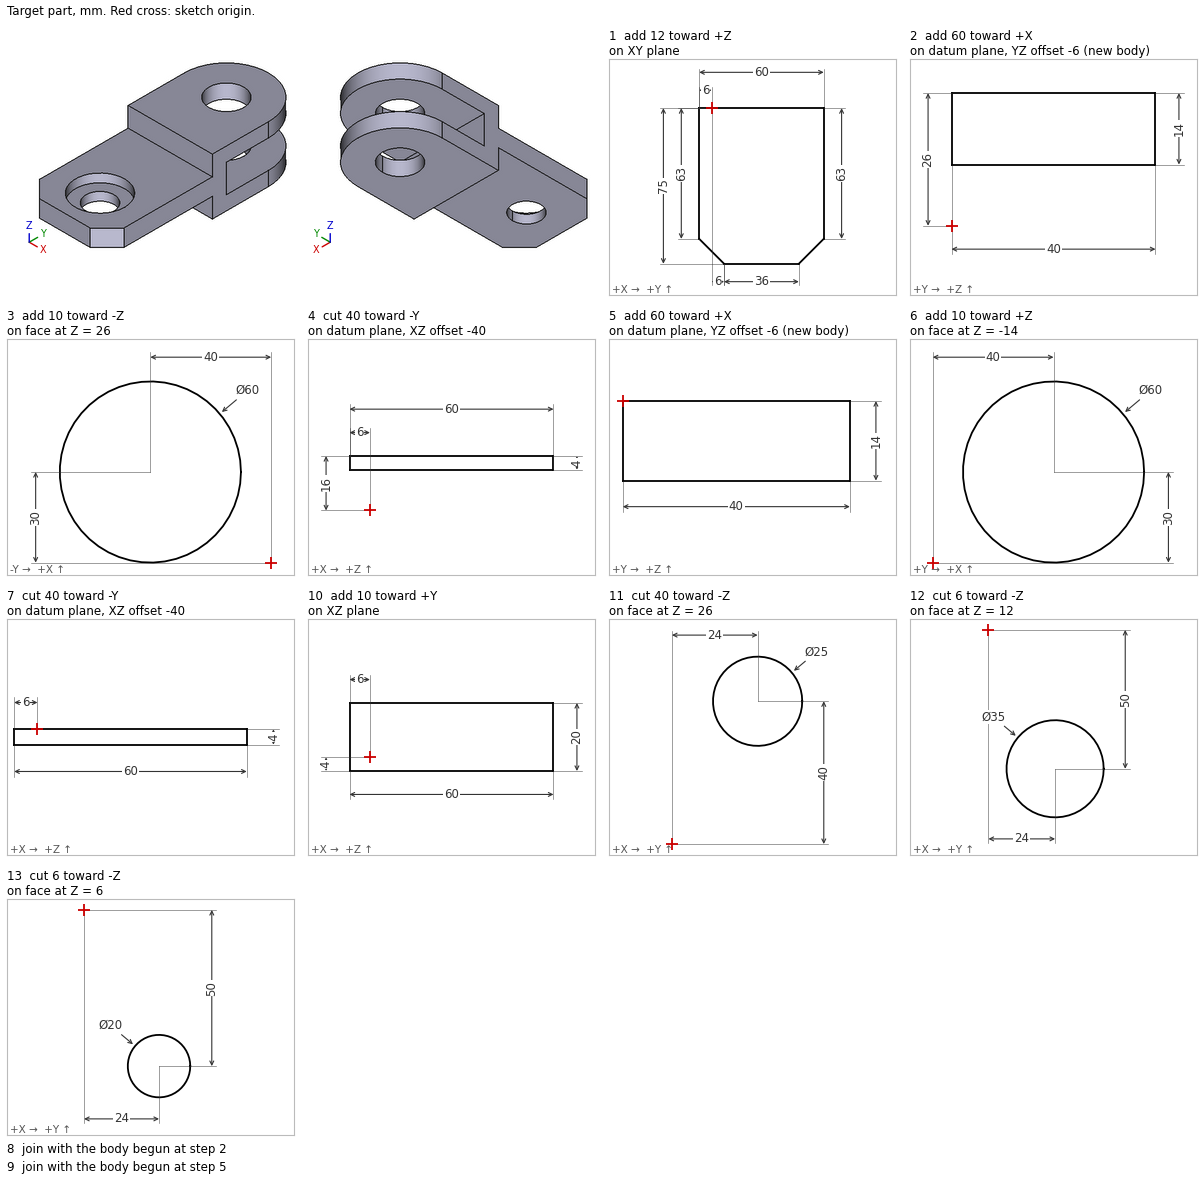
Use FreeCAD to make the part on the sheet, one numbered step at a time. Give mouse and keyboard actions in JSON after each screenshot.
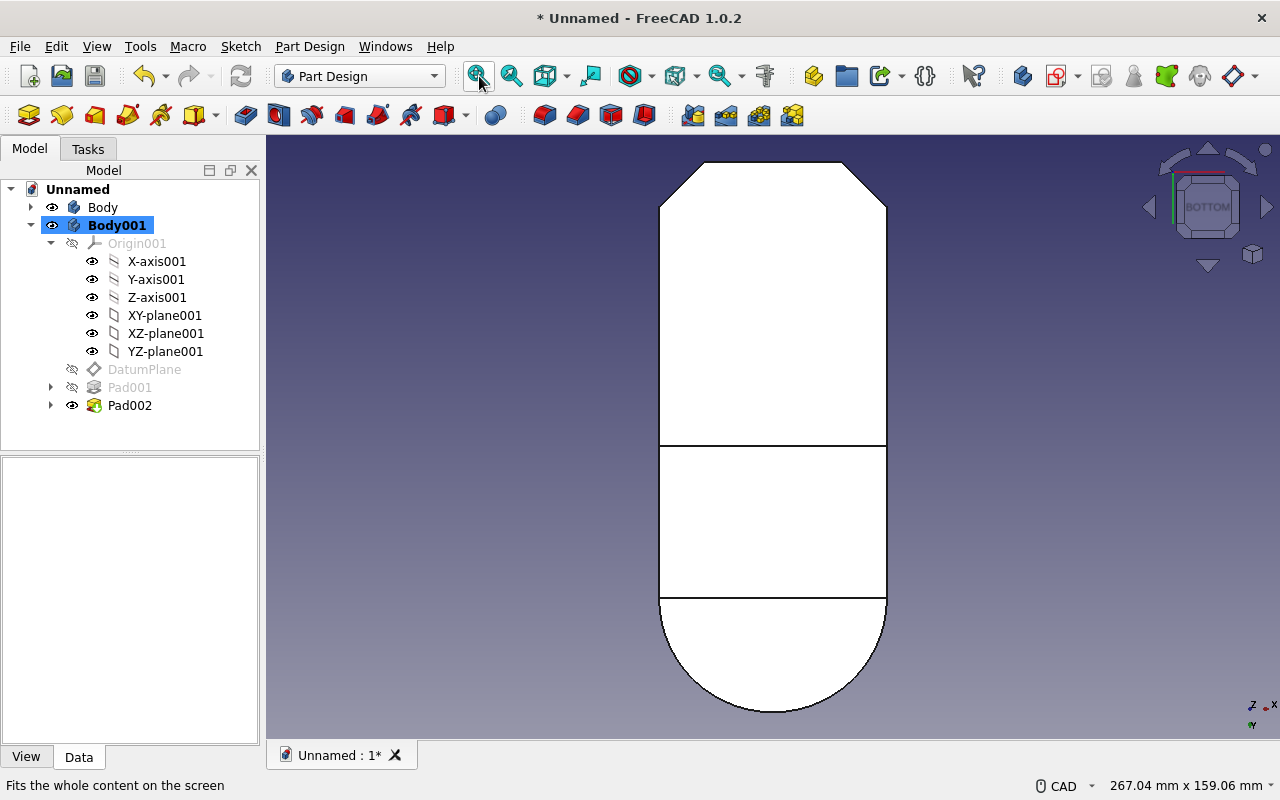
{"action": "key", "text": "3"}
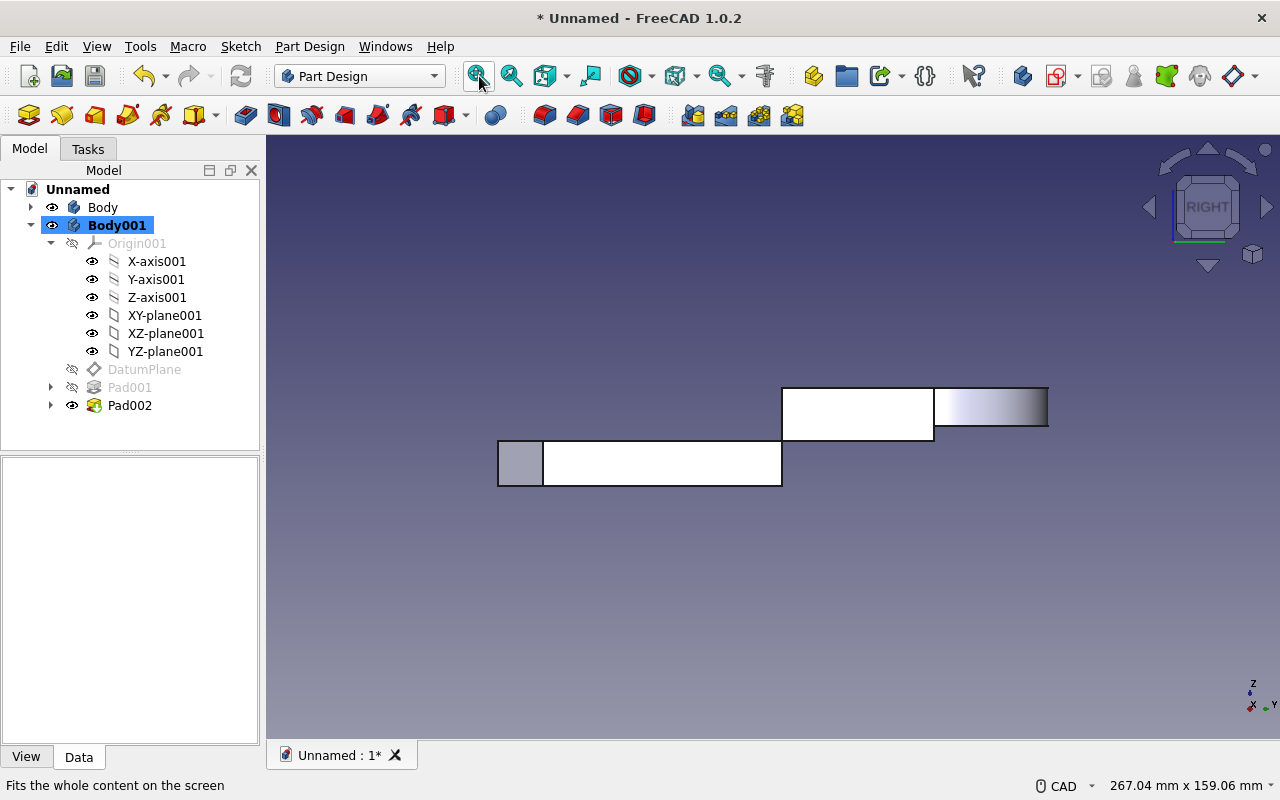
{"action": "left_click", "coordinate": [479, 76]}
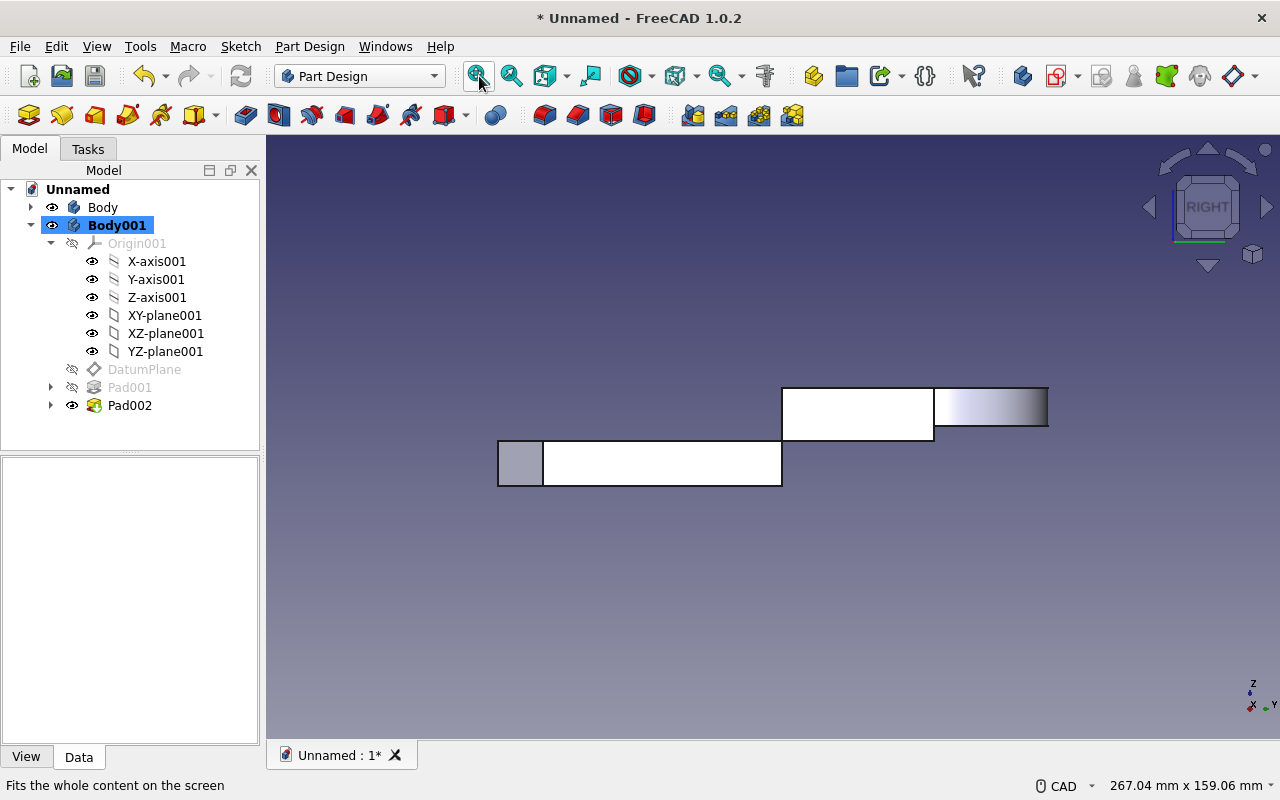
{"action": "left_click", "coordinate": [137, 333]}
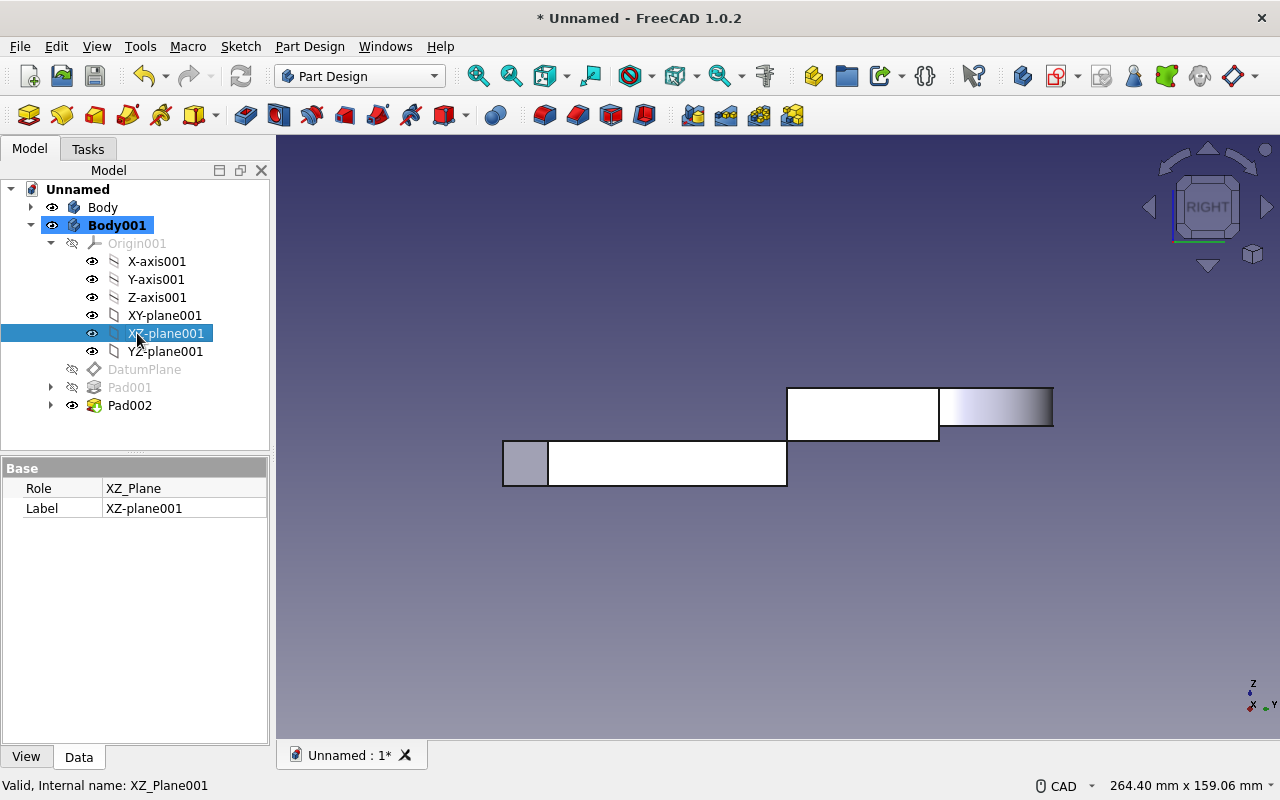
{"action": "left_click", "coordinate": [1232, 76]}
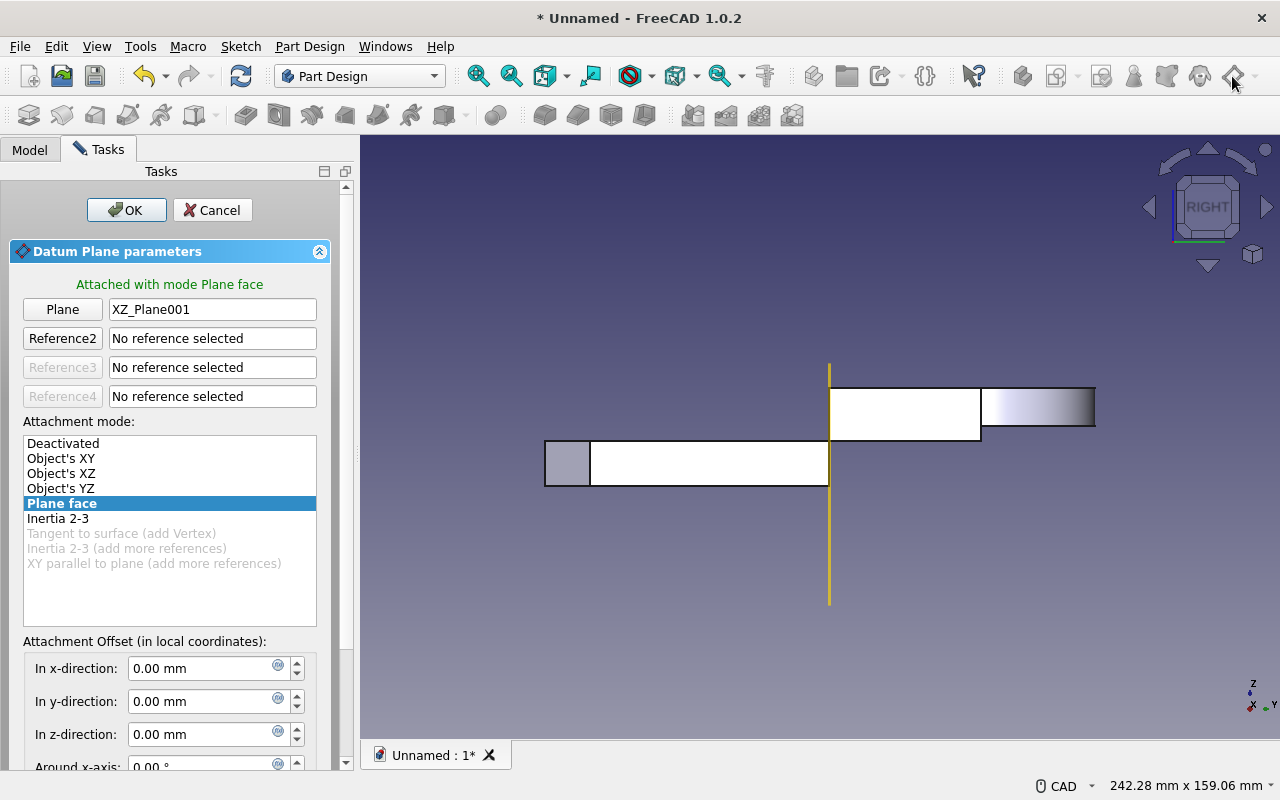
{"action": "triple_click", "coordinate": [210, 734]}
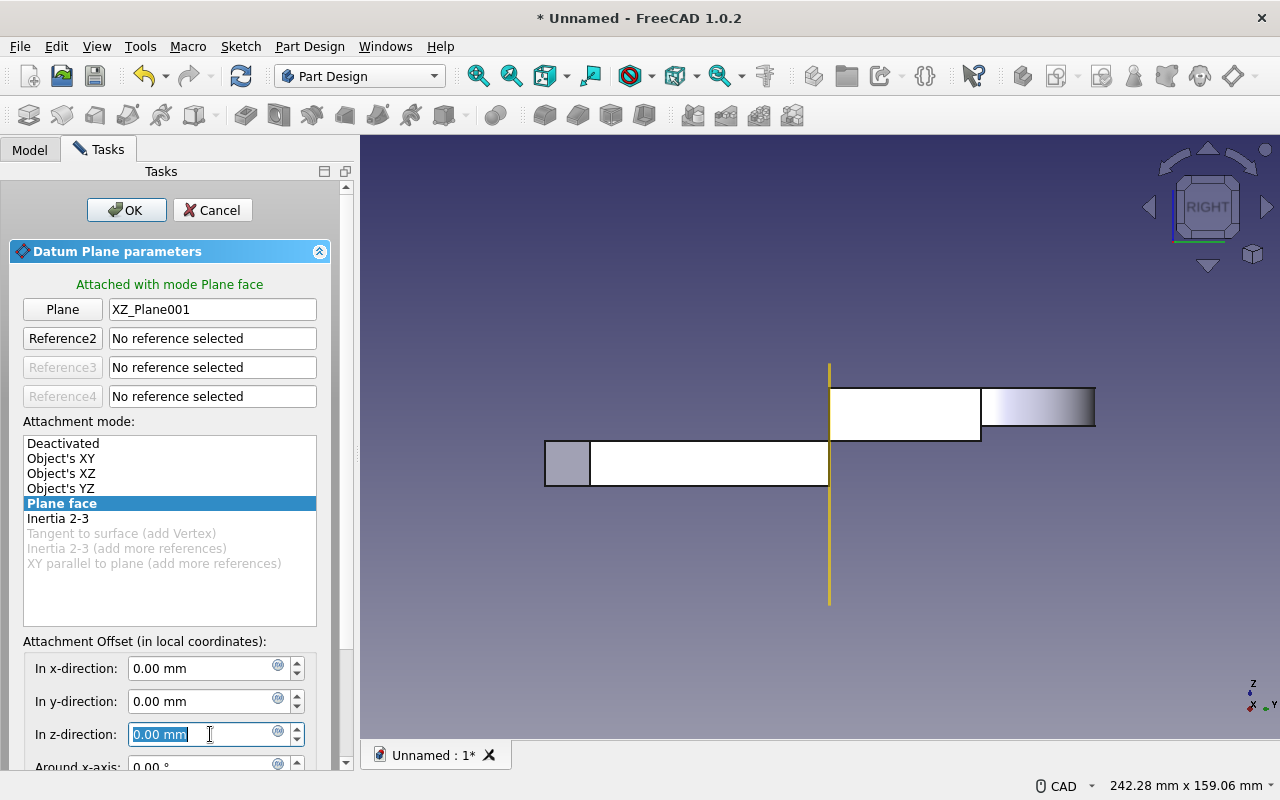
{"action": "type", "text": "-40"}
{"action": "key", "text": "Tab"}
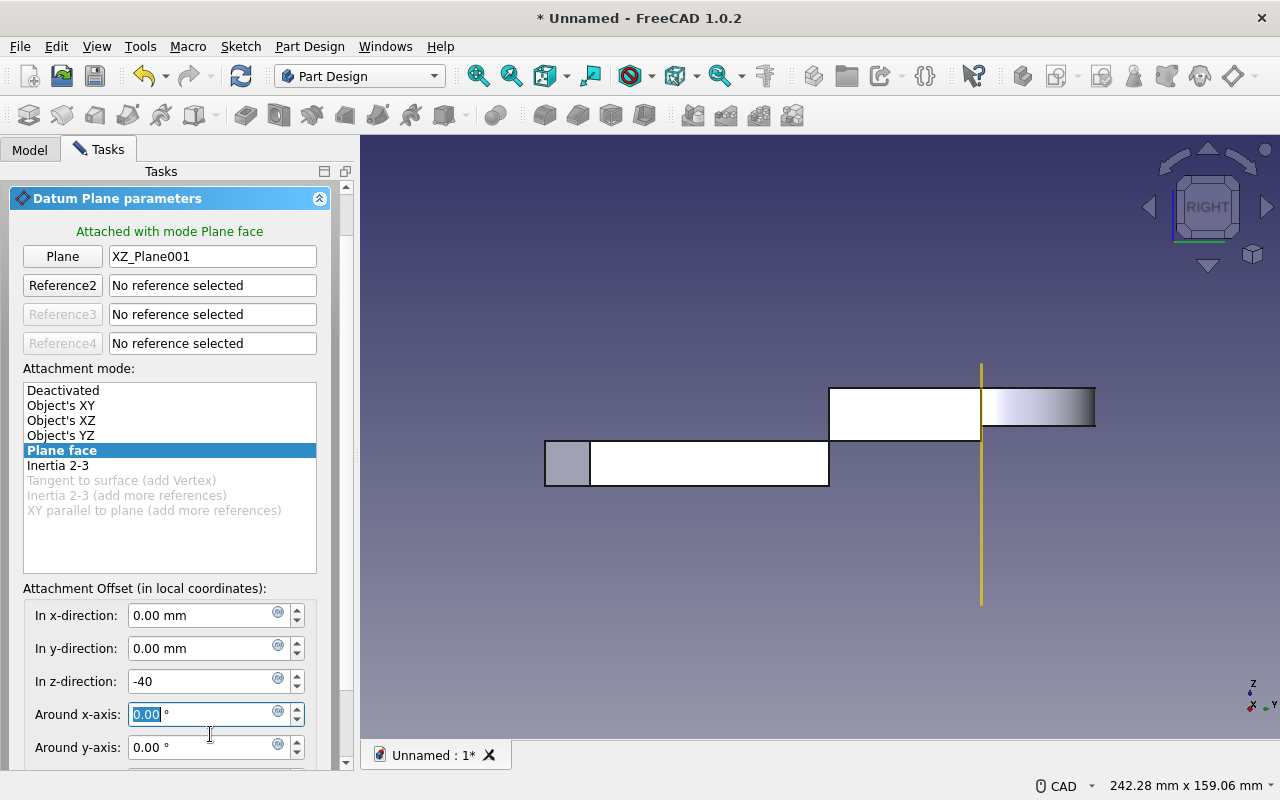
{"action": "scroll", "coordinate": [346, 476], "scroll_direction": "up", "scroll_amount": 2}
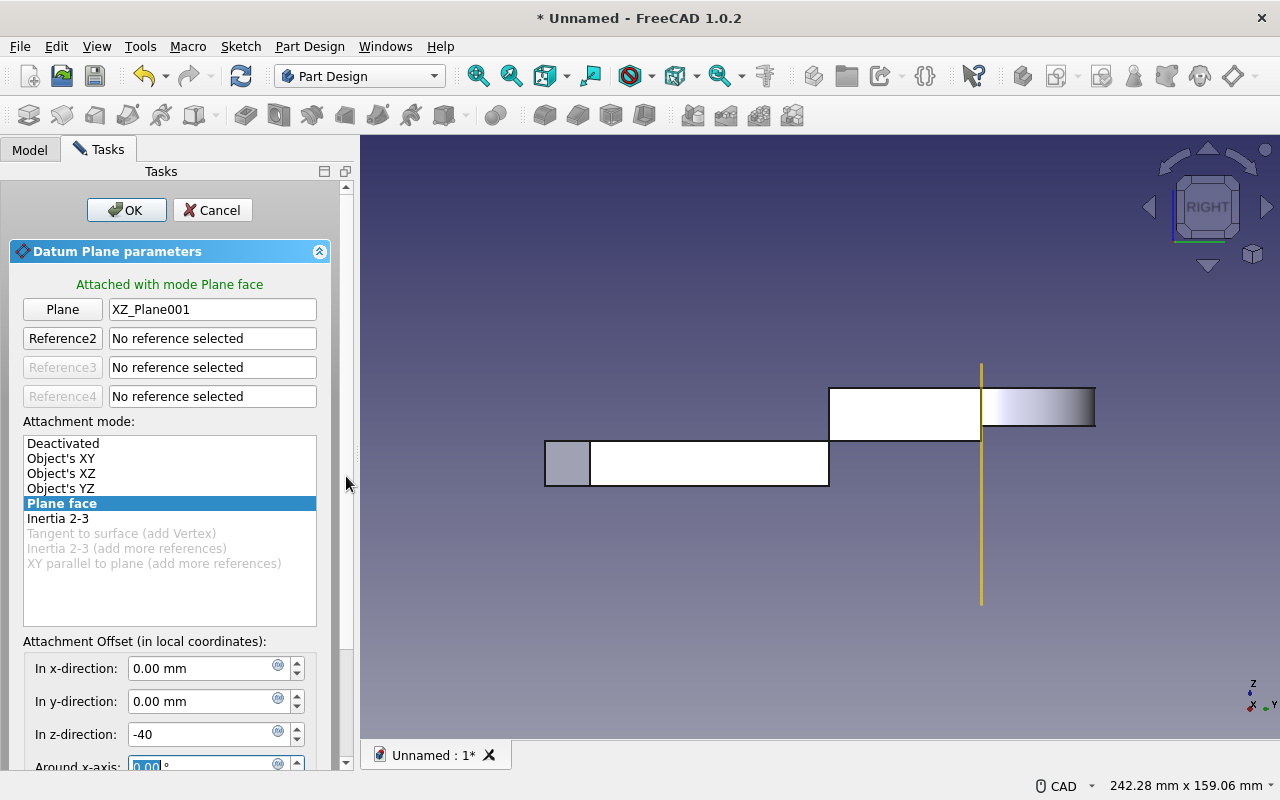
{"action": "left_click", "coordinate": [127, 210]}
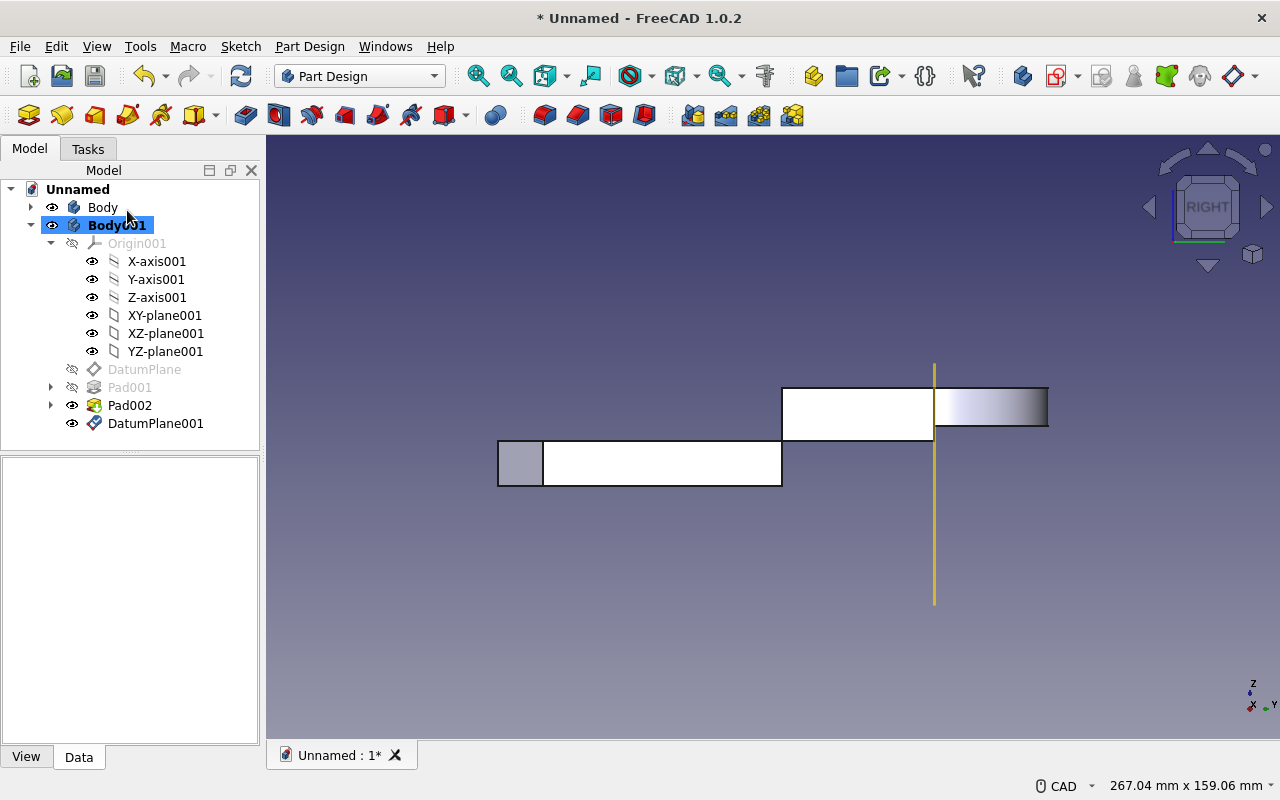
{"action": "left_click", "coordinate": [117, 423]}